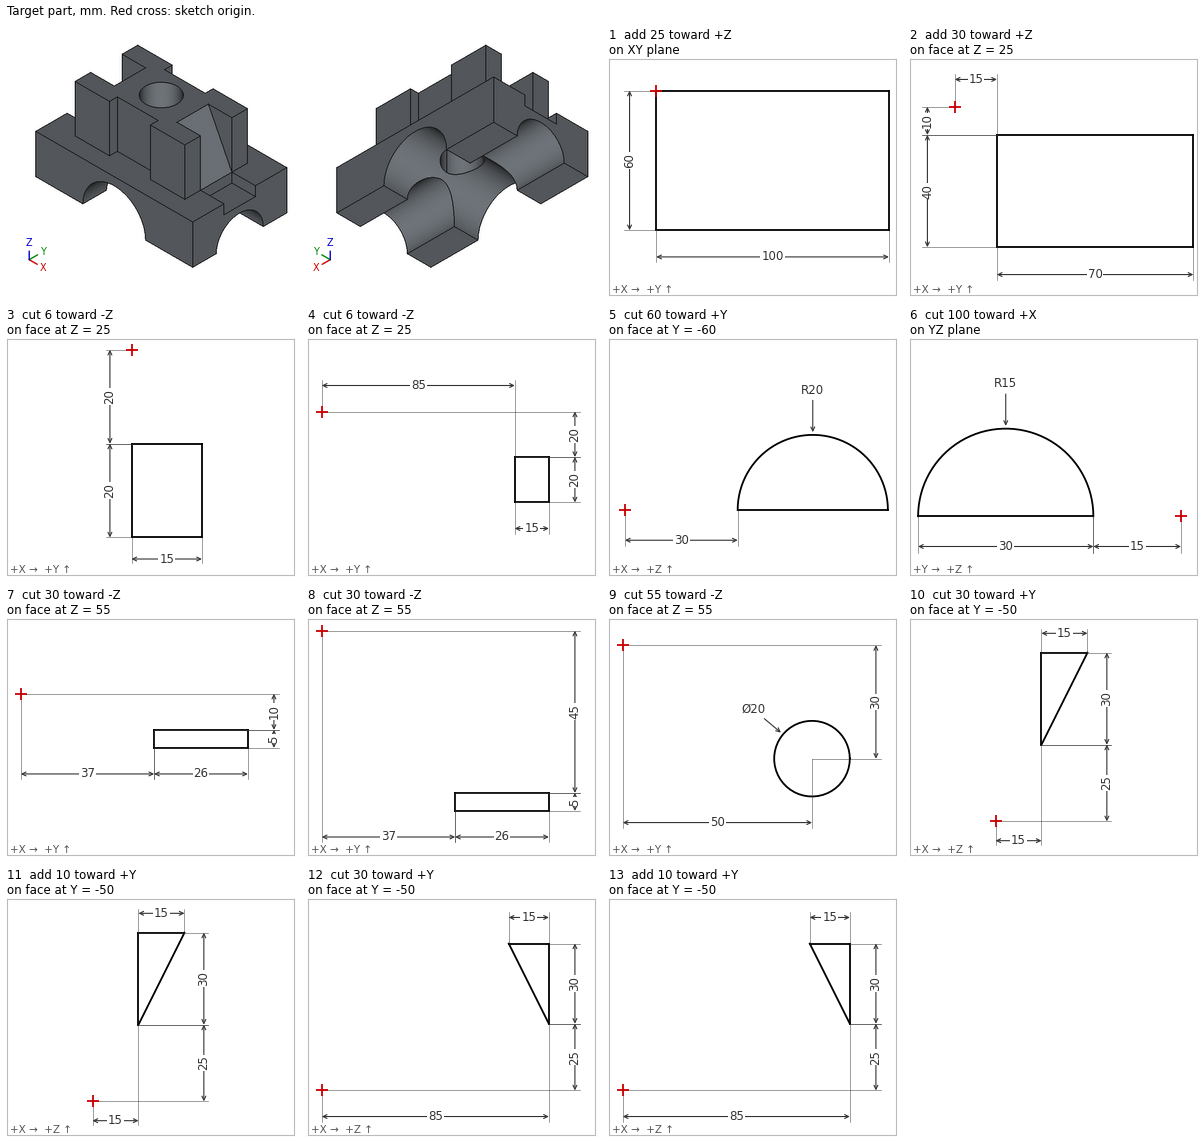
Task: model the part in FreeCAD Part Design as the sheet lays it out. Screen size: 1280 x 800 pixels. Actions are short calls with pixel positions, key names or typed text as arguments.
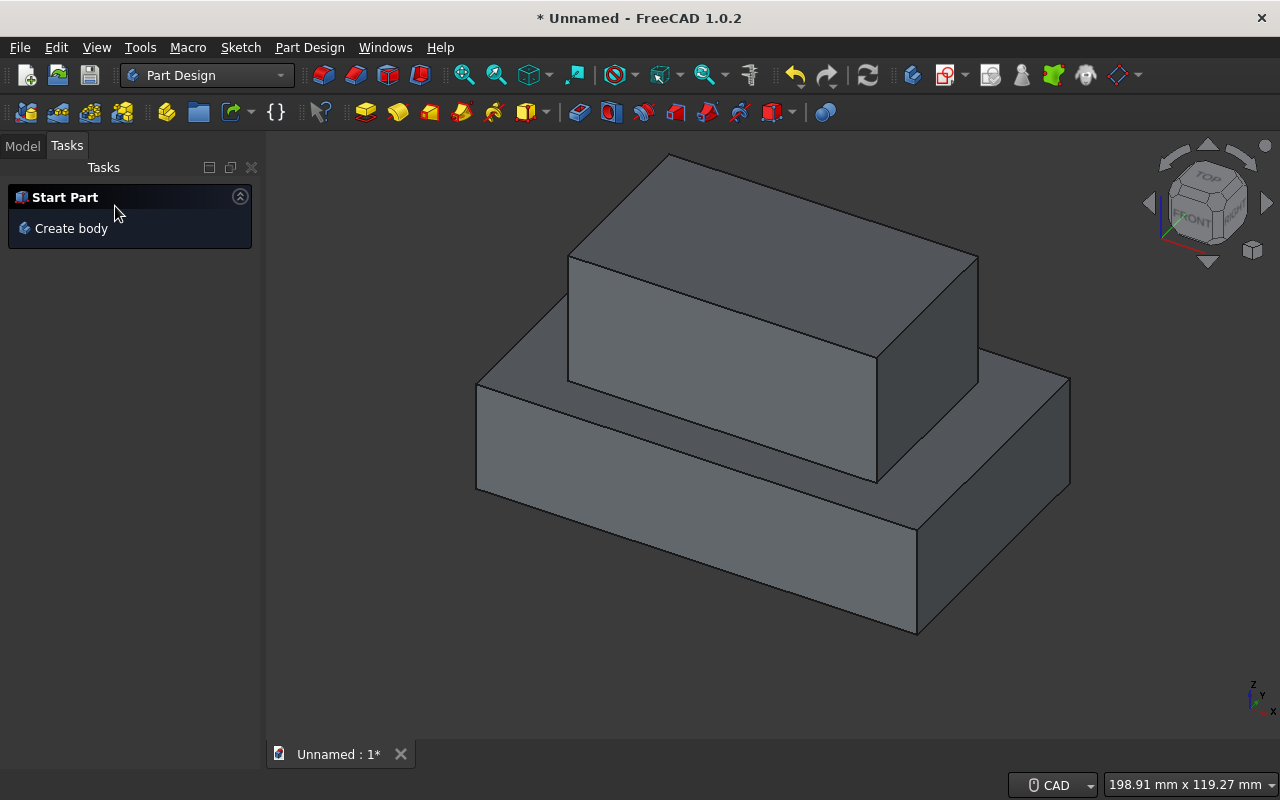
click(466, 76)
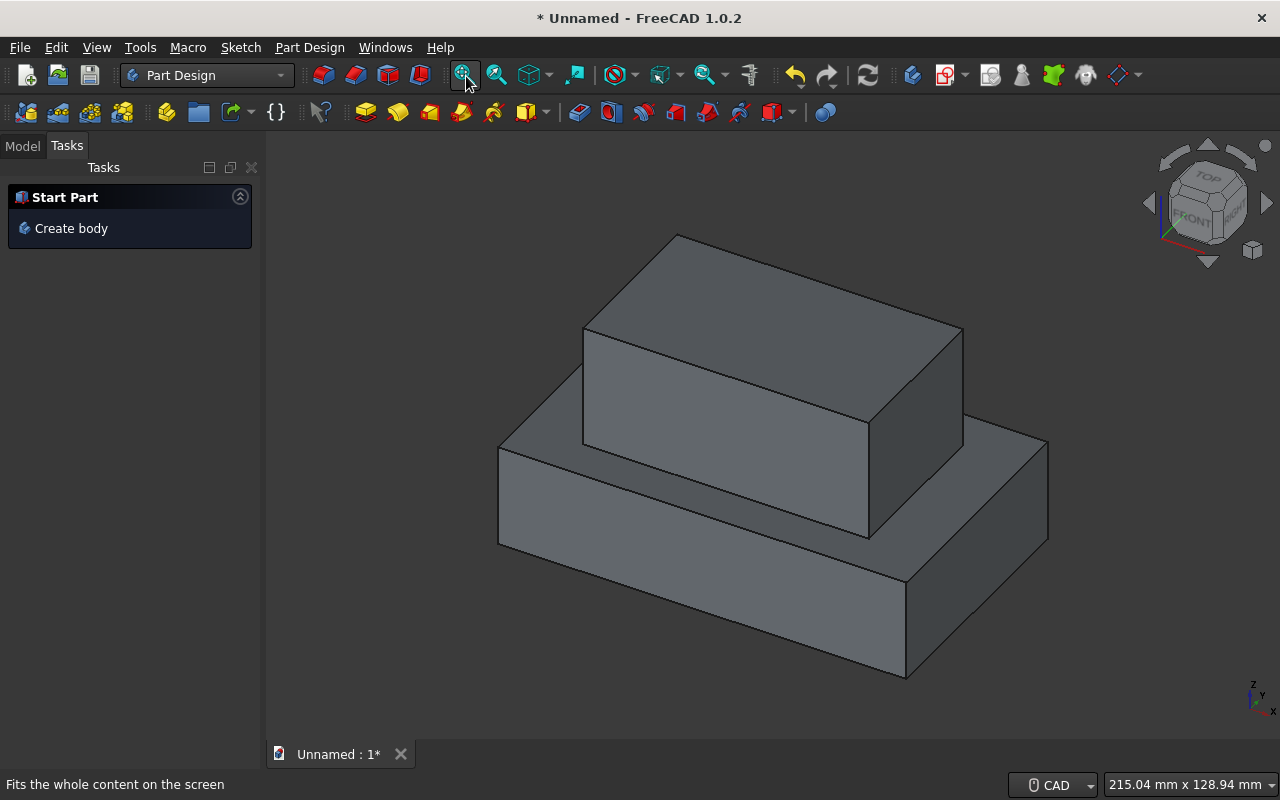
click(558, 426)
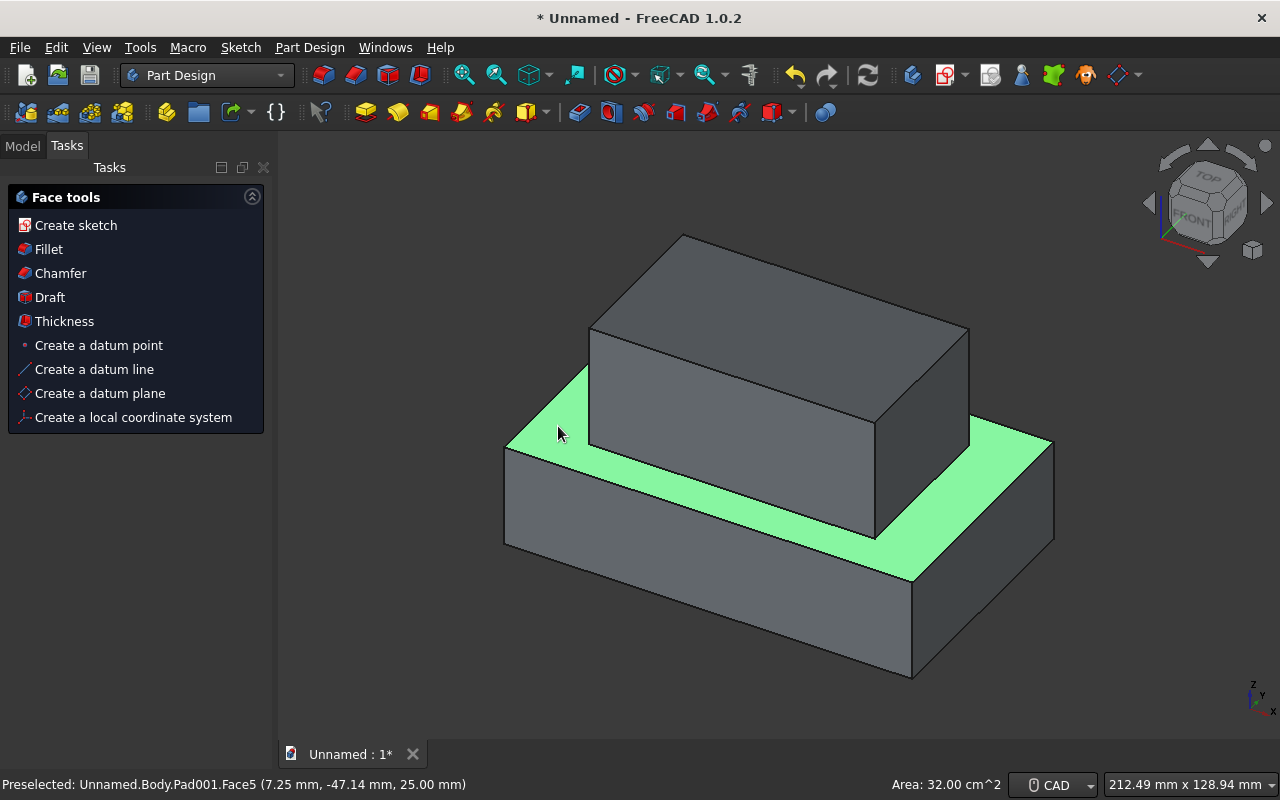
click(946, 76)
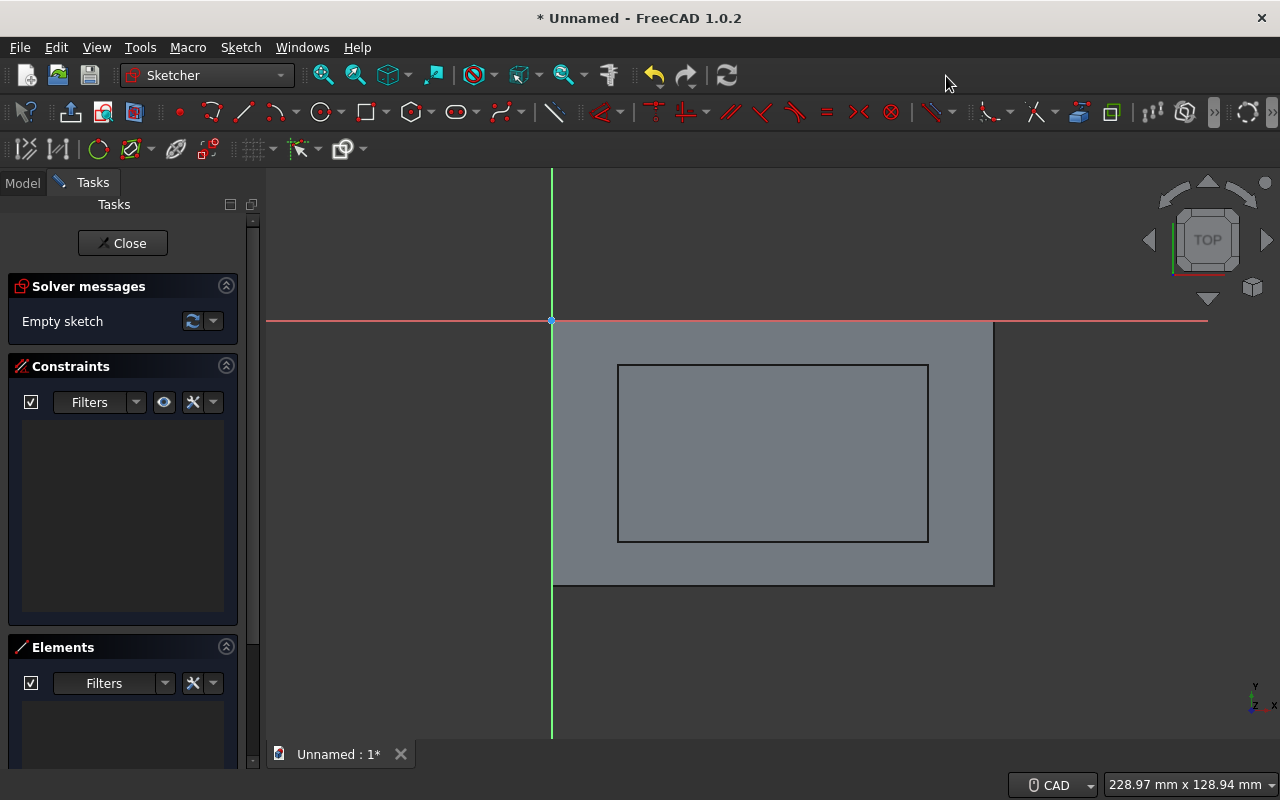
key(q)
key(s)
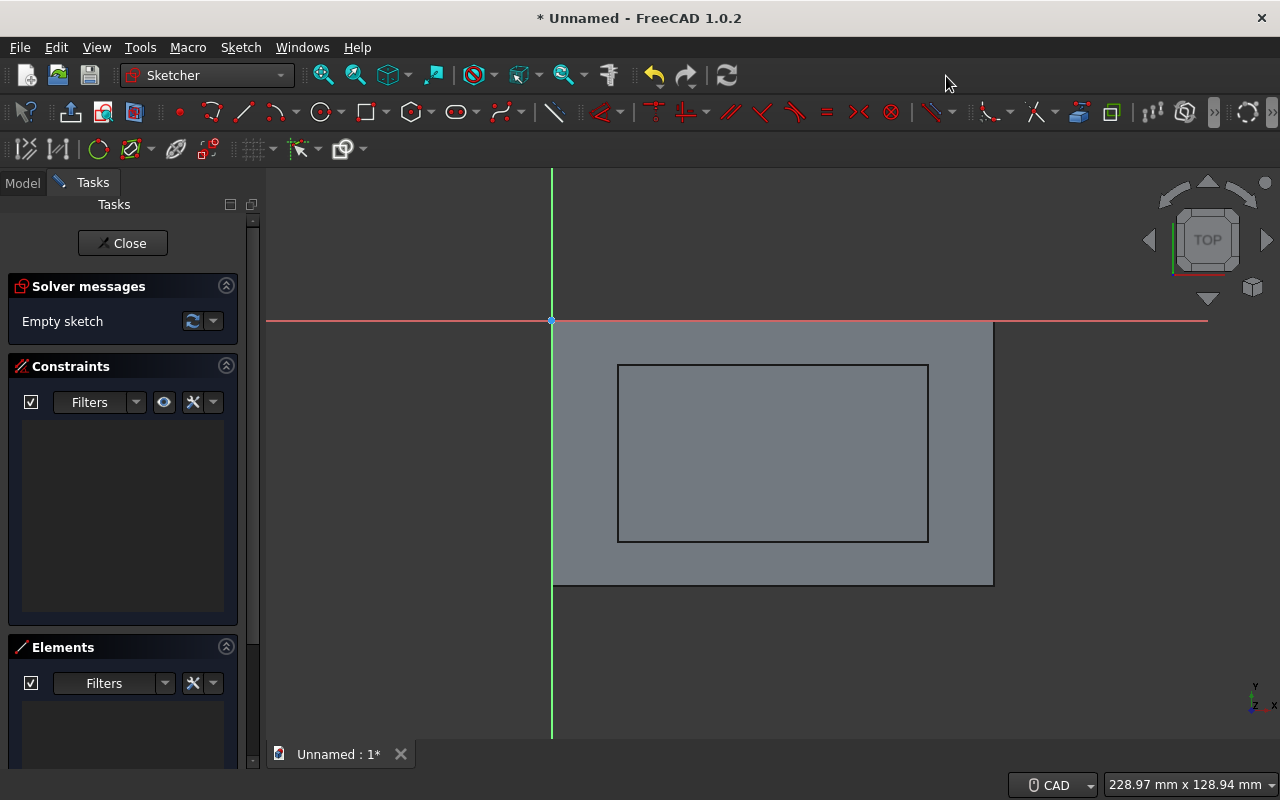
scroll(487, 373, up, 4)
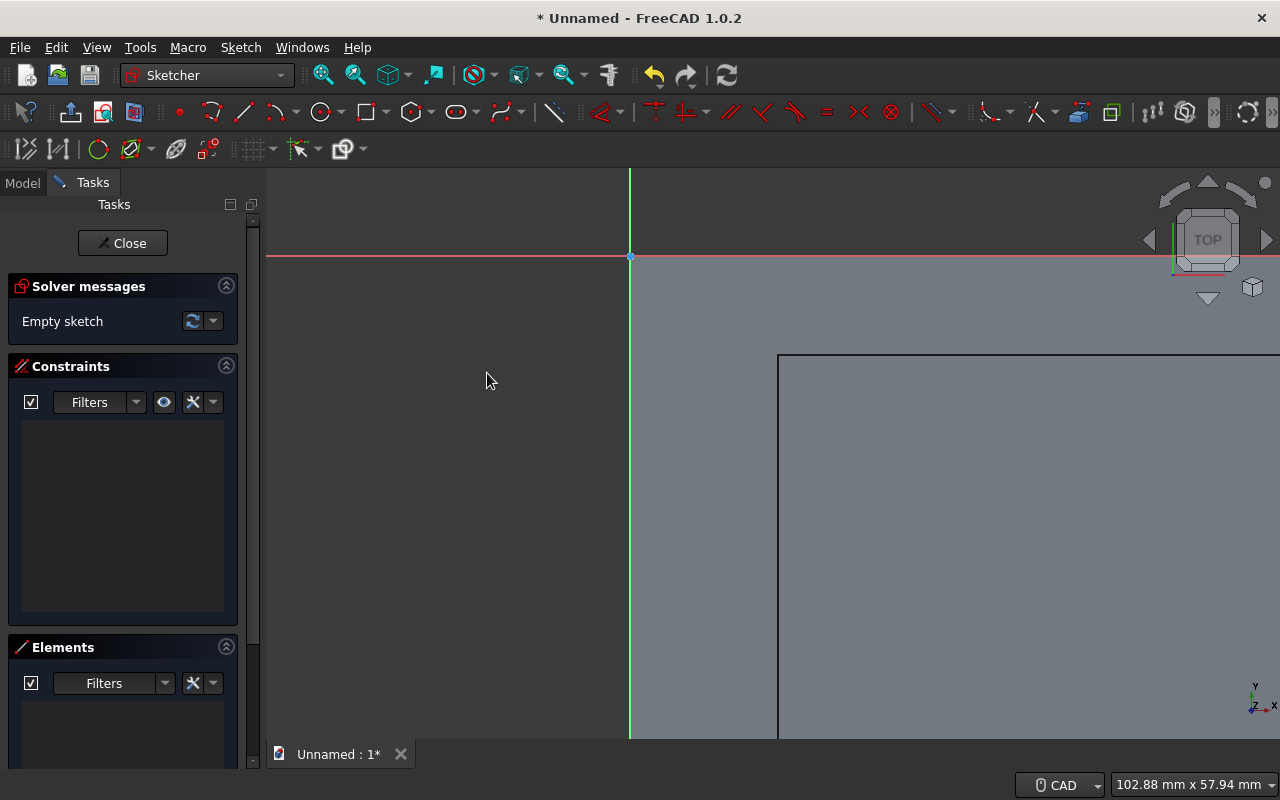
key(g)
key(r)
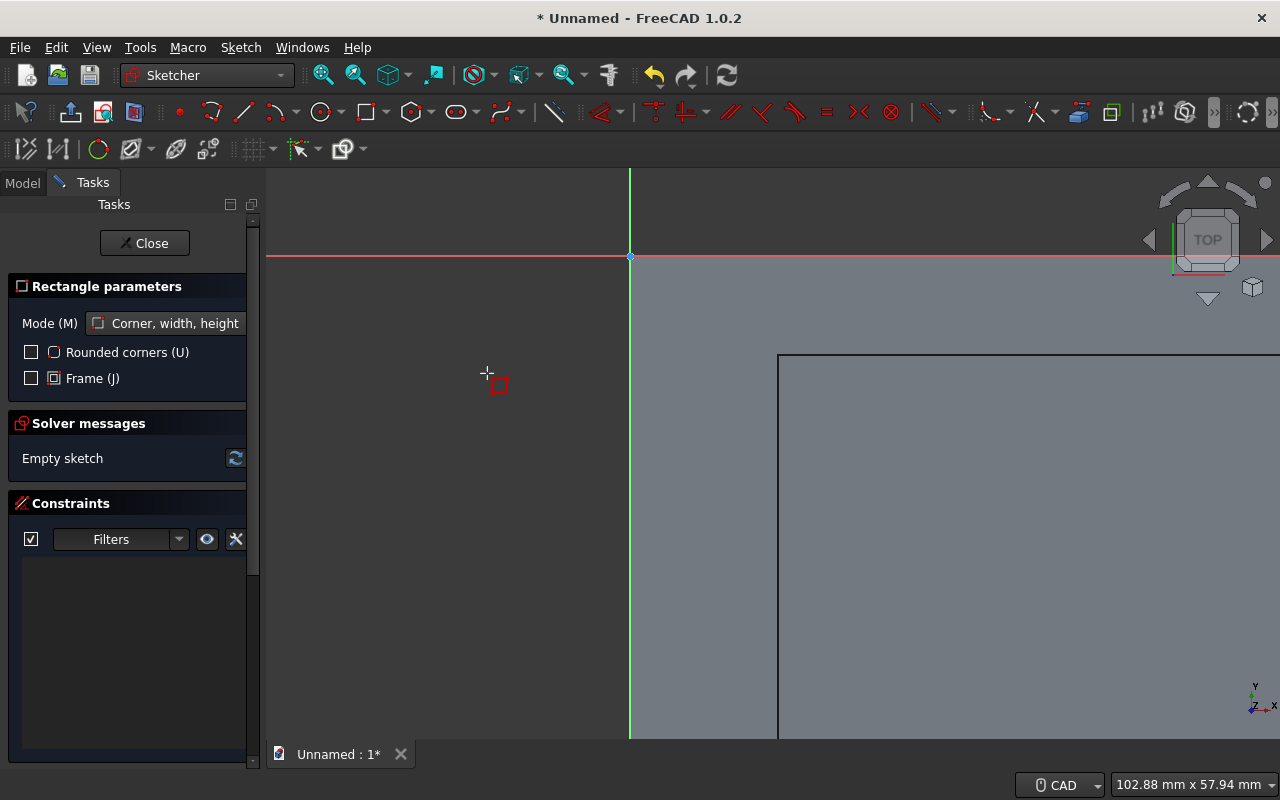
click(630, 453)
click(778, 650)
key(Escape)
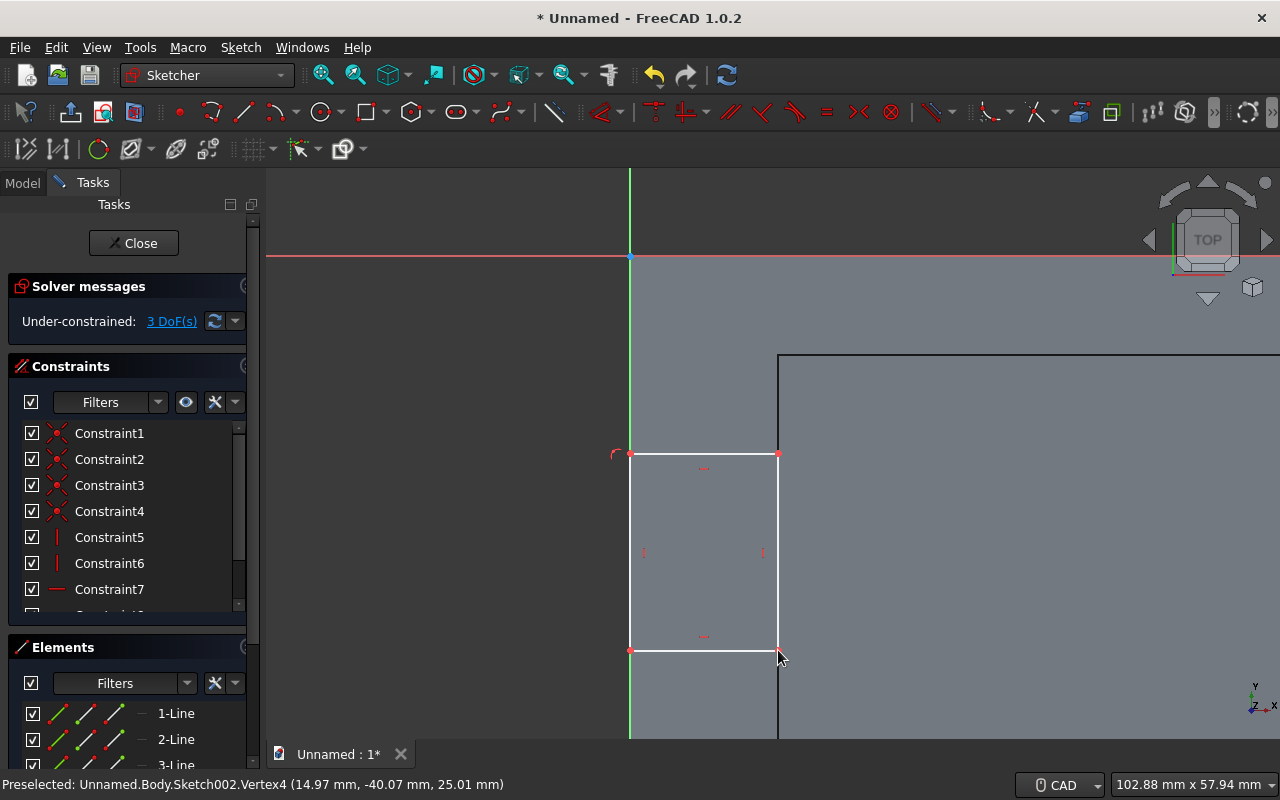
key(d)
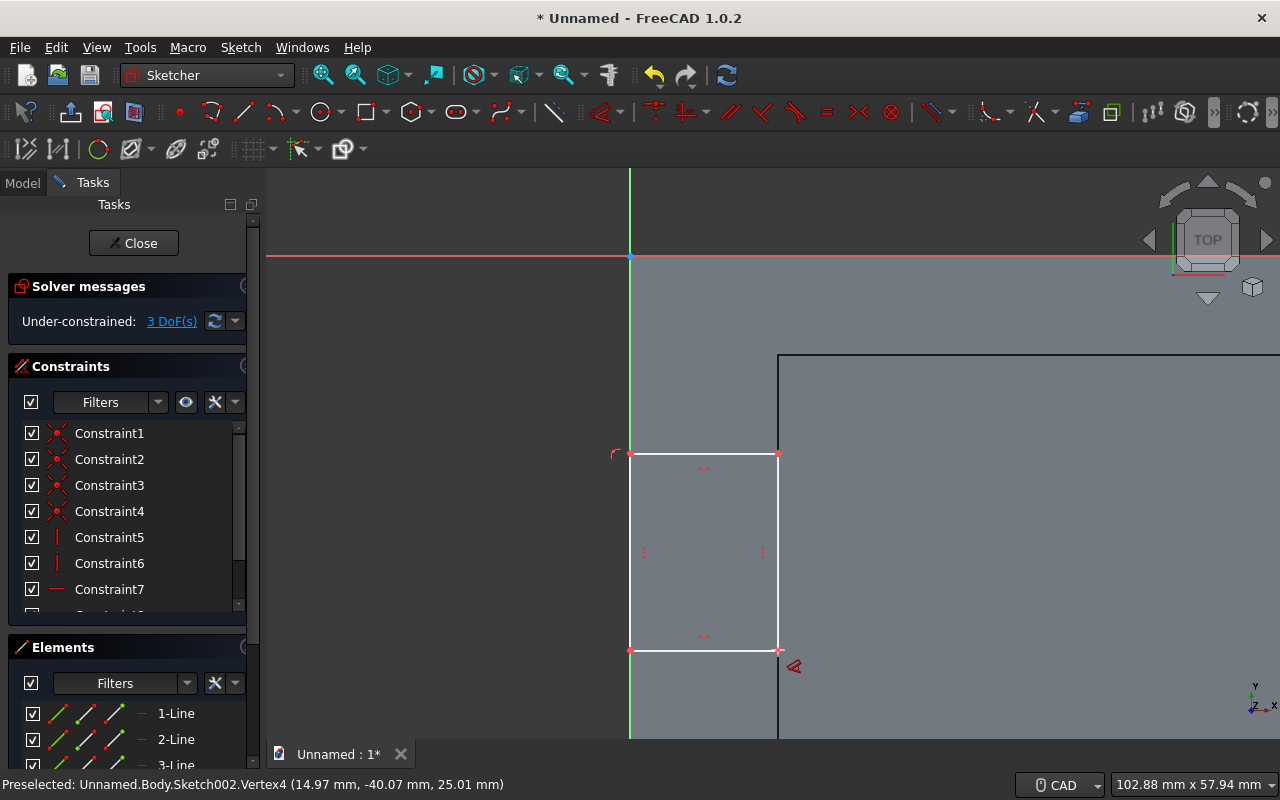
click(630, 513)
click(596, 553)